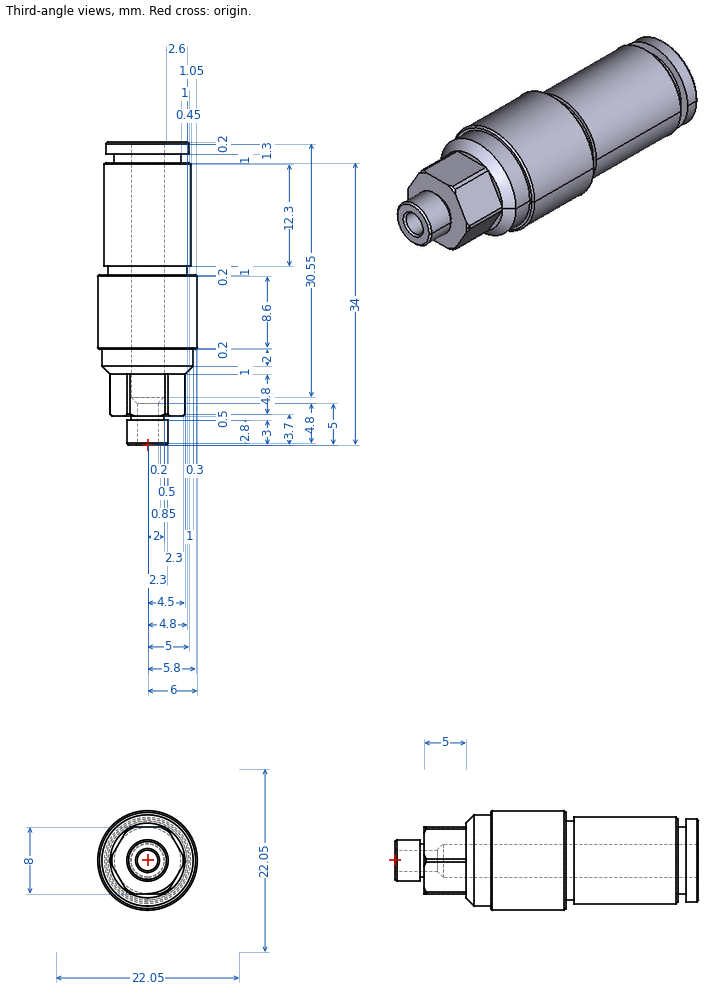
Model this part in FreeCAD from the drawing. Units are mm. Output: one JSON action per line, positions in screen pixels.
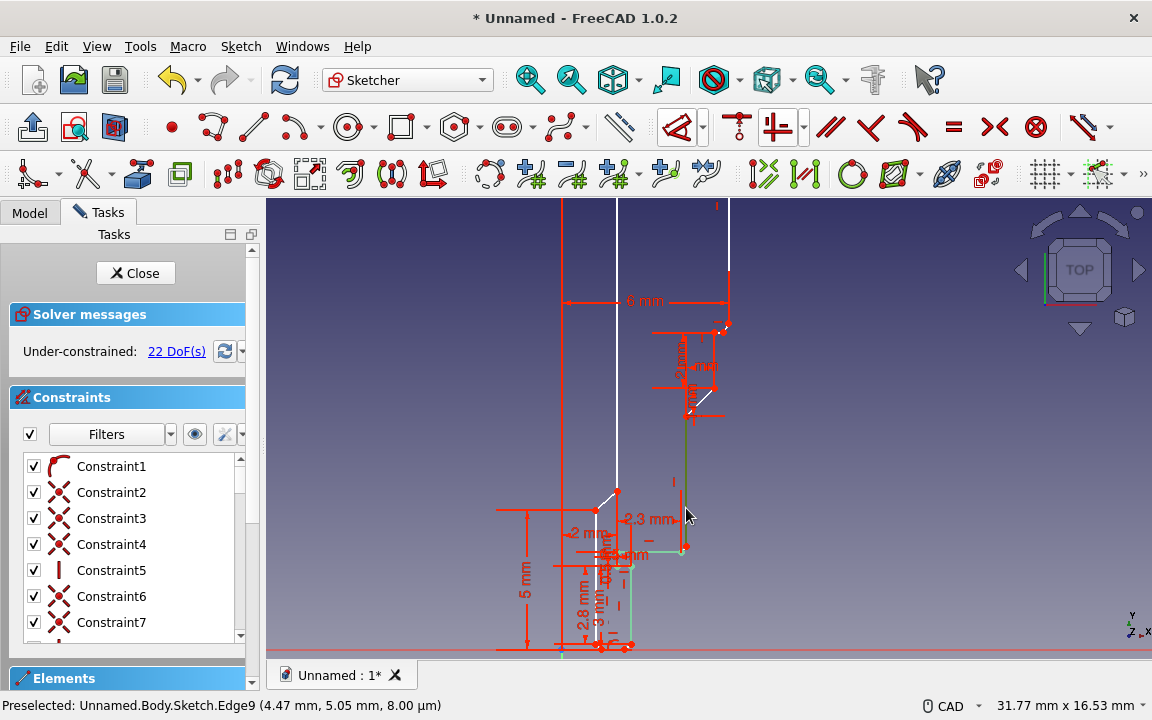
{"action": "left_click", "coordinate": [702, 128]}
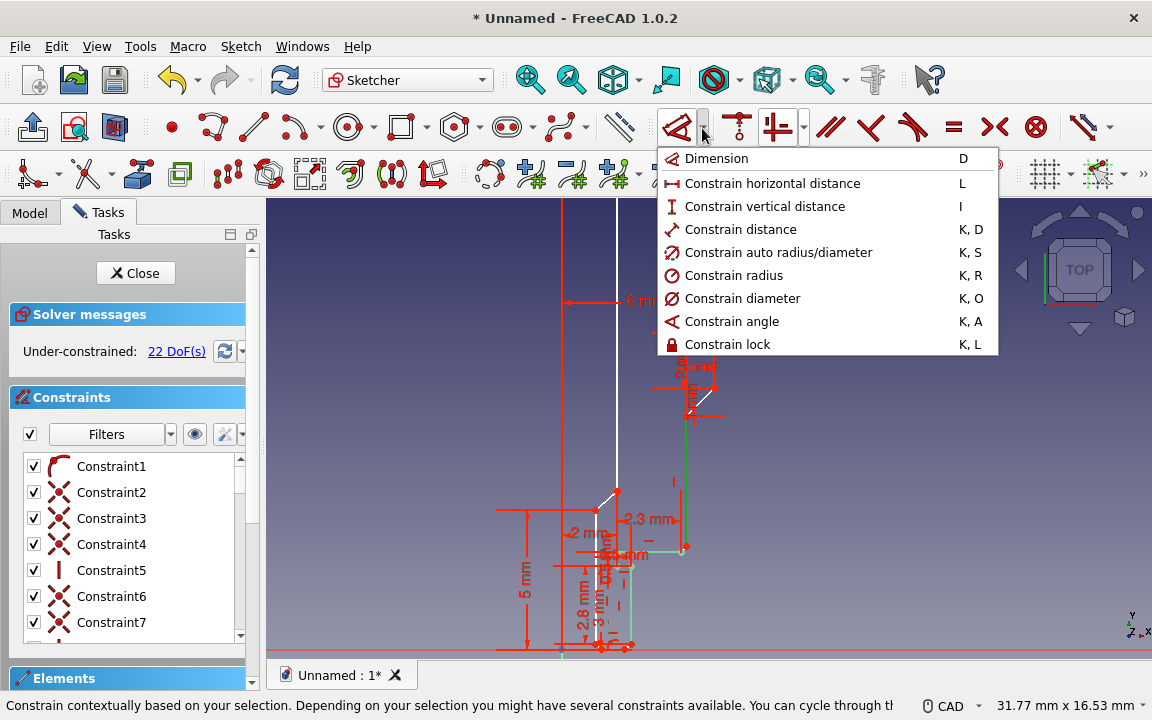
{"action": "left_click", "coordinate": [828, 206]}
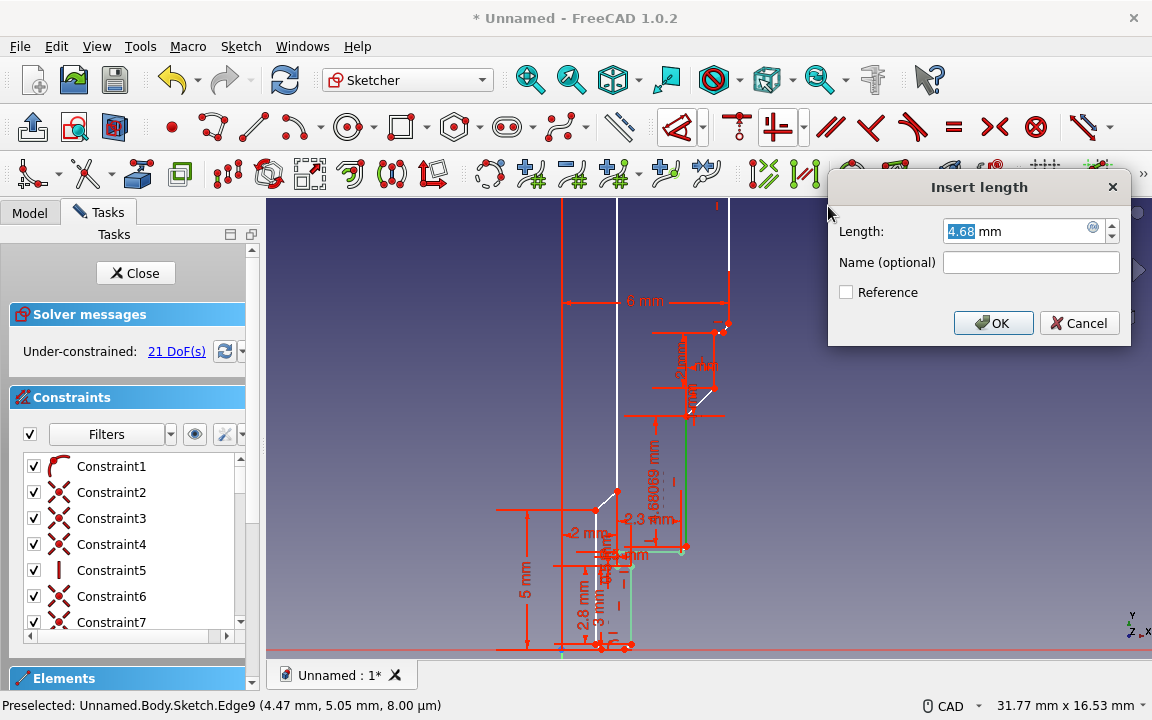
{"action": "type", "text": "4.8"}
{"action": "key", "text": "Return"}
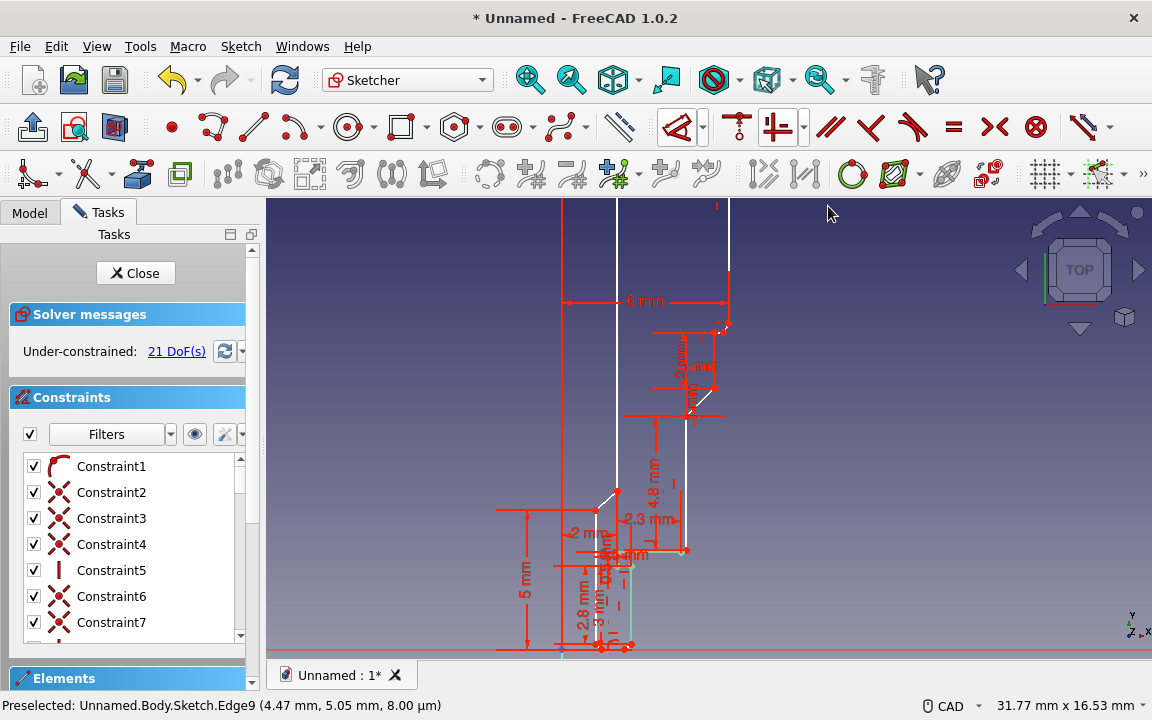
{"action": "scroll", "coordinate": [719, 333], "scroll_direction": "up", "scroll_amount": 8}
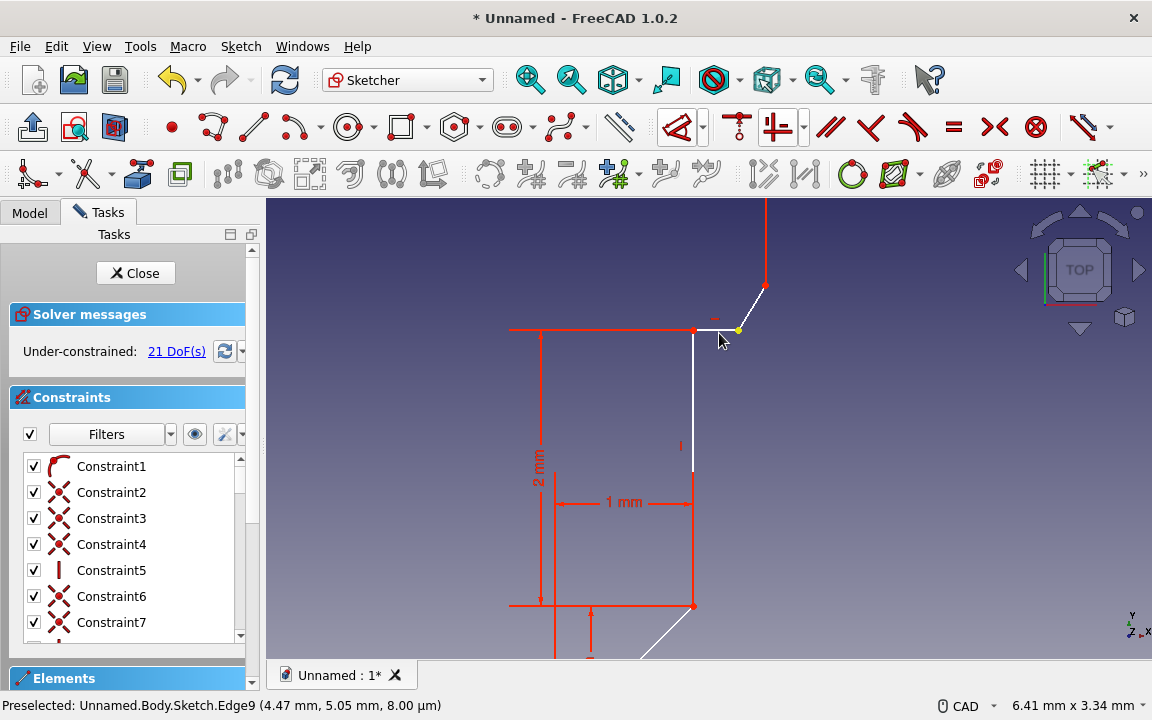
{"action": "left_click", "coordinate": [716, 330]}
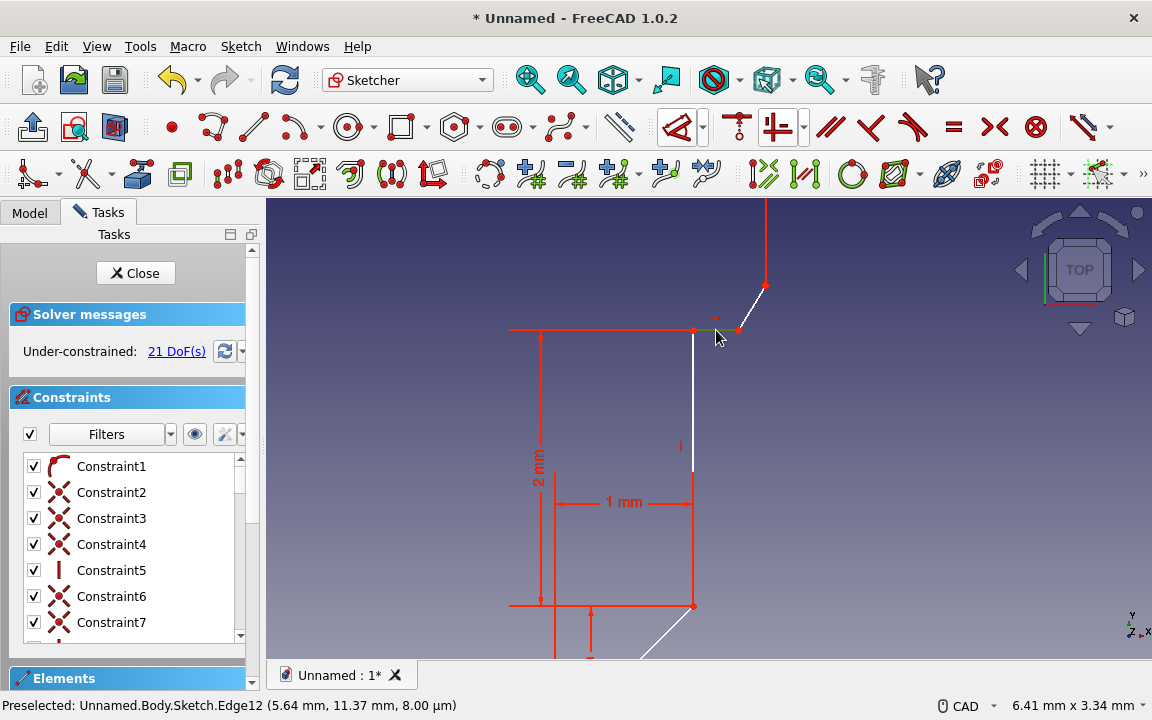
{"action": "key", "text": "l"}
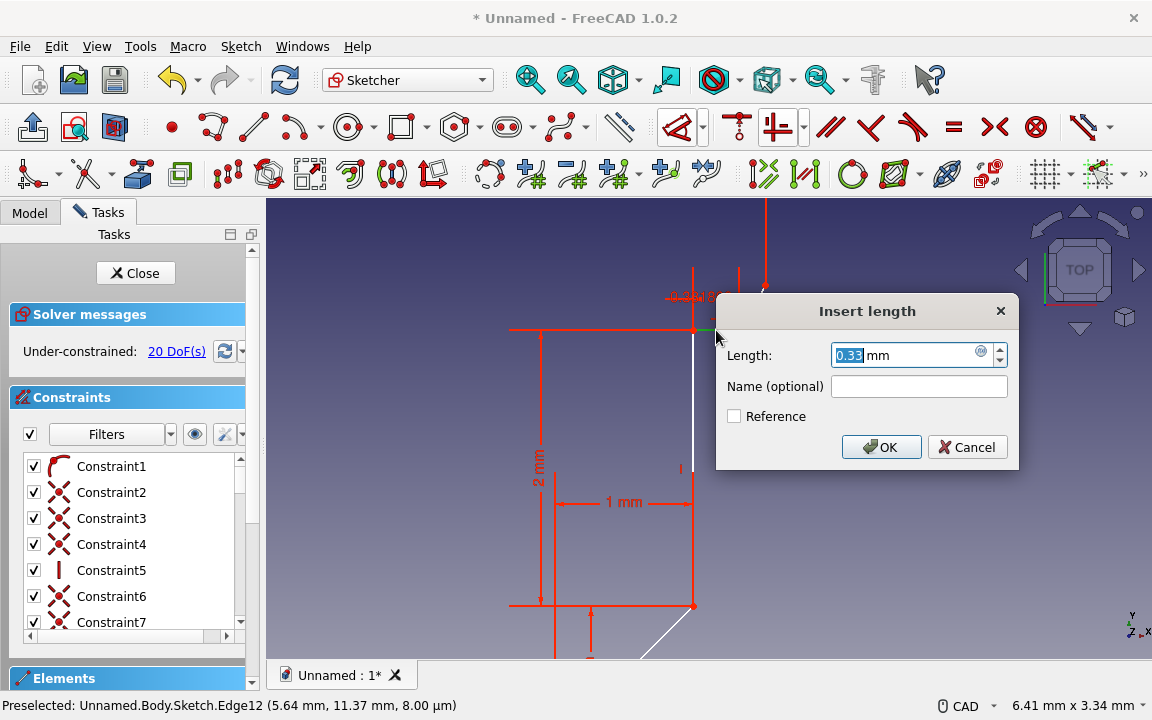
{"action": "type", "text": "0.3"}
{"action": "key", "text": "Return"}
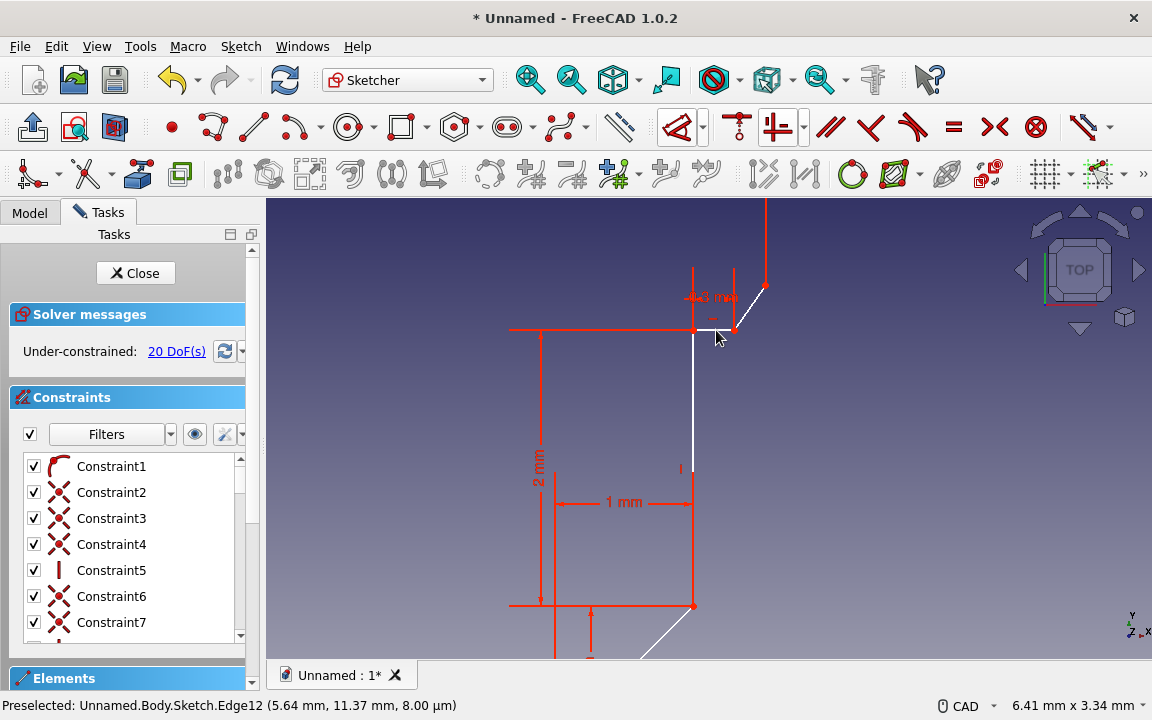
{"action": "scroll", "coordinate": [659, 496], "scroll_direction": "down", "scroll_amount": 14}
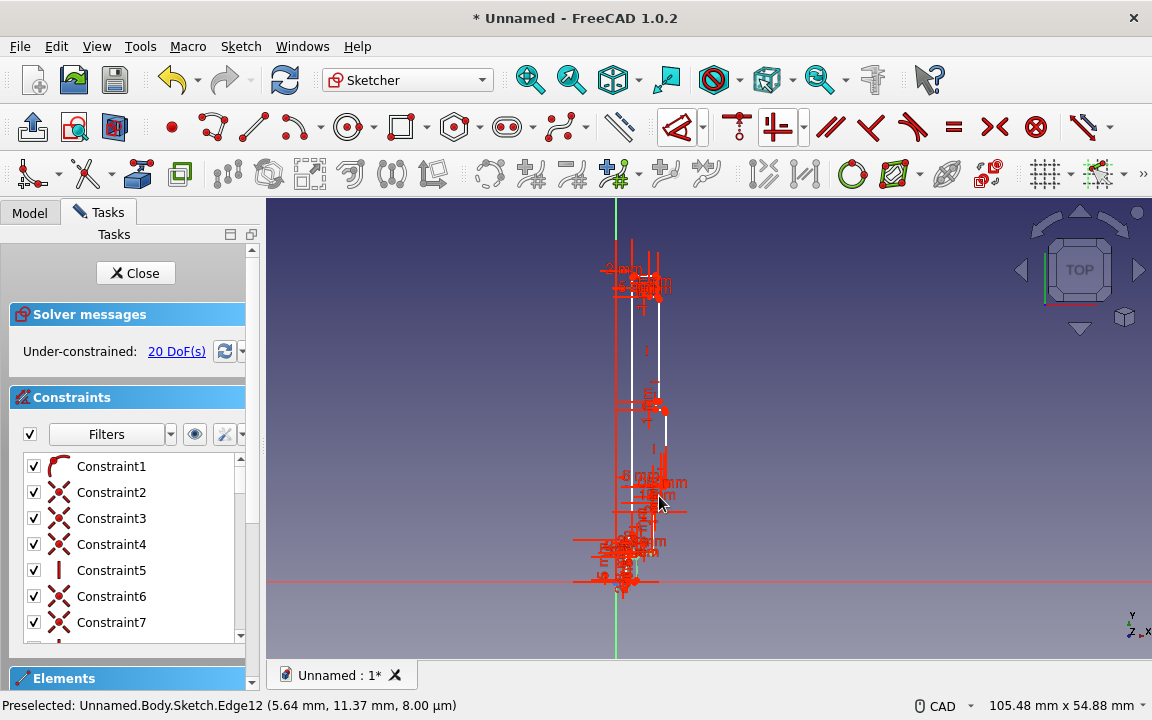
{"action": "left_click", "coordinate": [666, 434]}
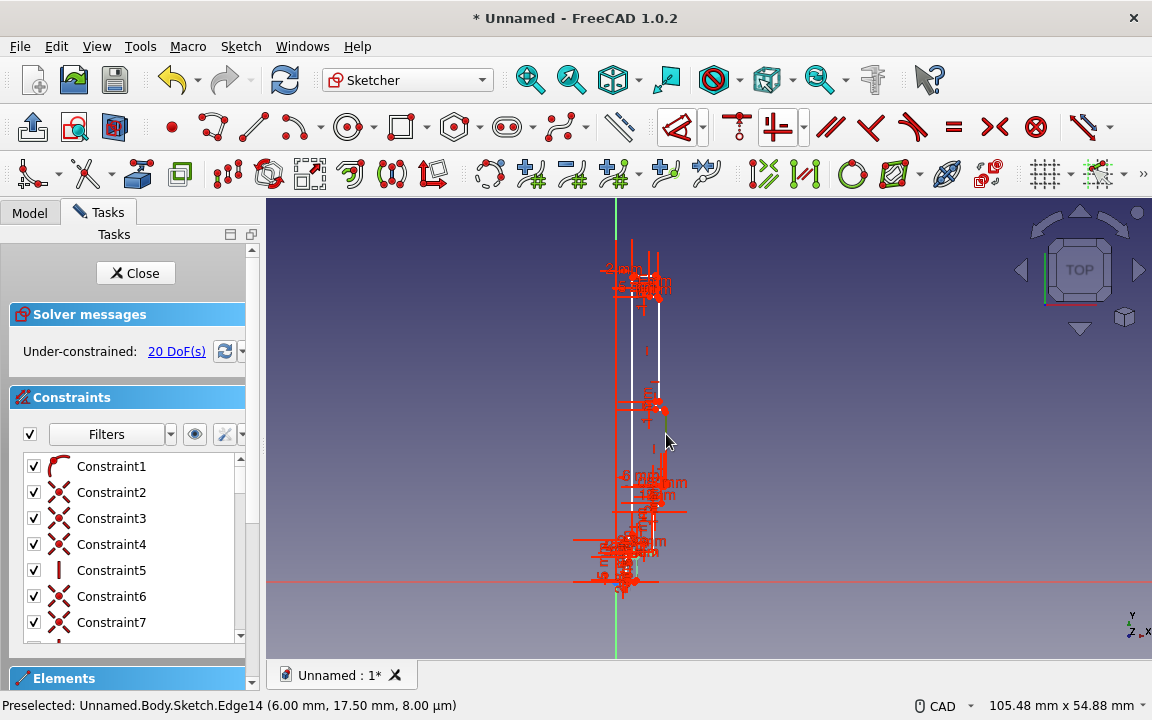
{"action": "key", "text": "i"}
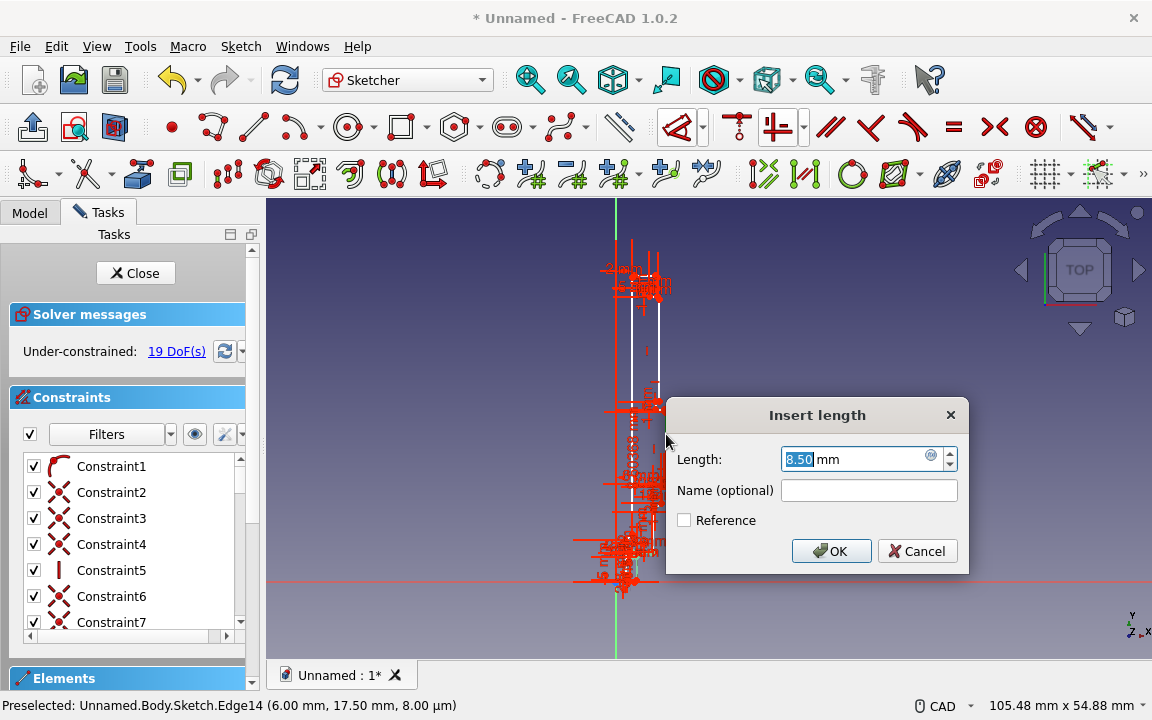
{"action": "type", "text": "8.6"}
{"action": "key", "text": "Return"}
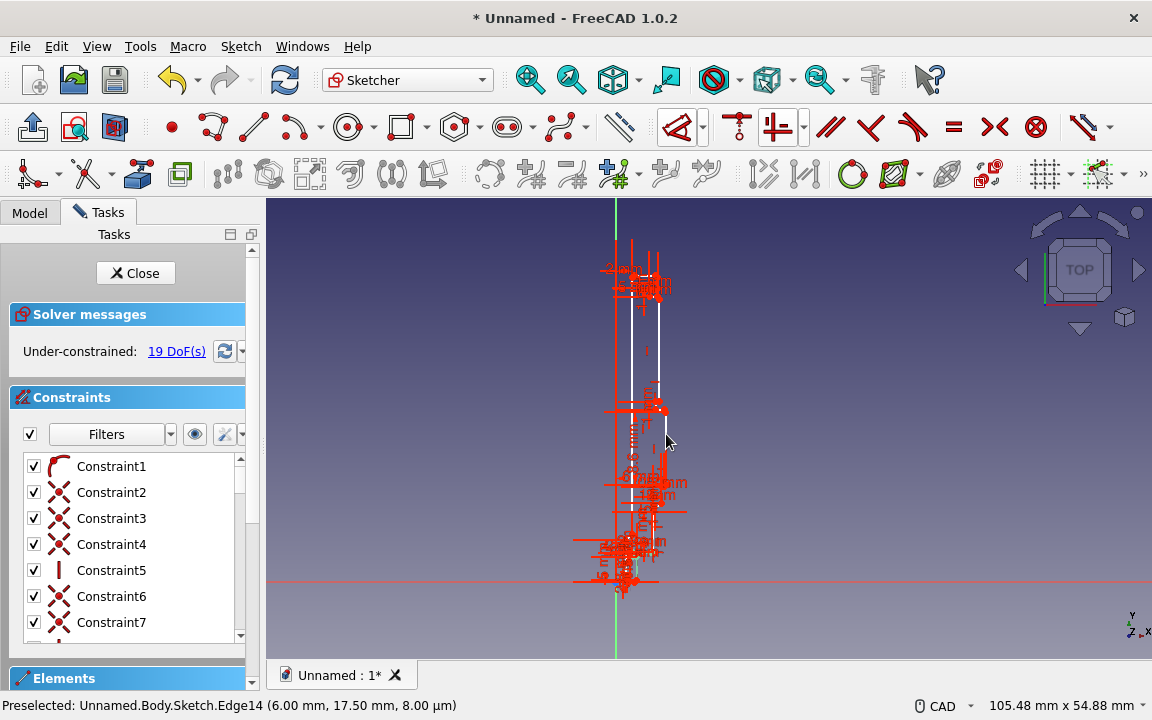
{"action": "scroll", "coordinate": [658, 283], "scroll_direction": "up", "scroll_amount": 7}